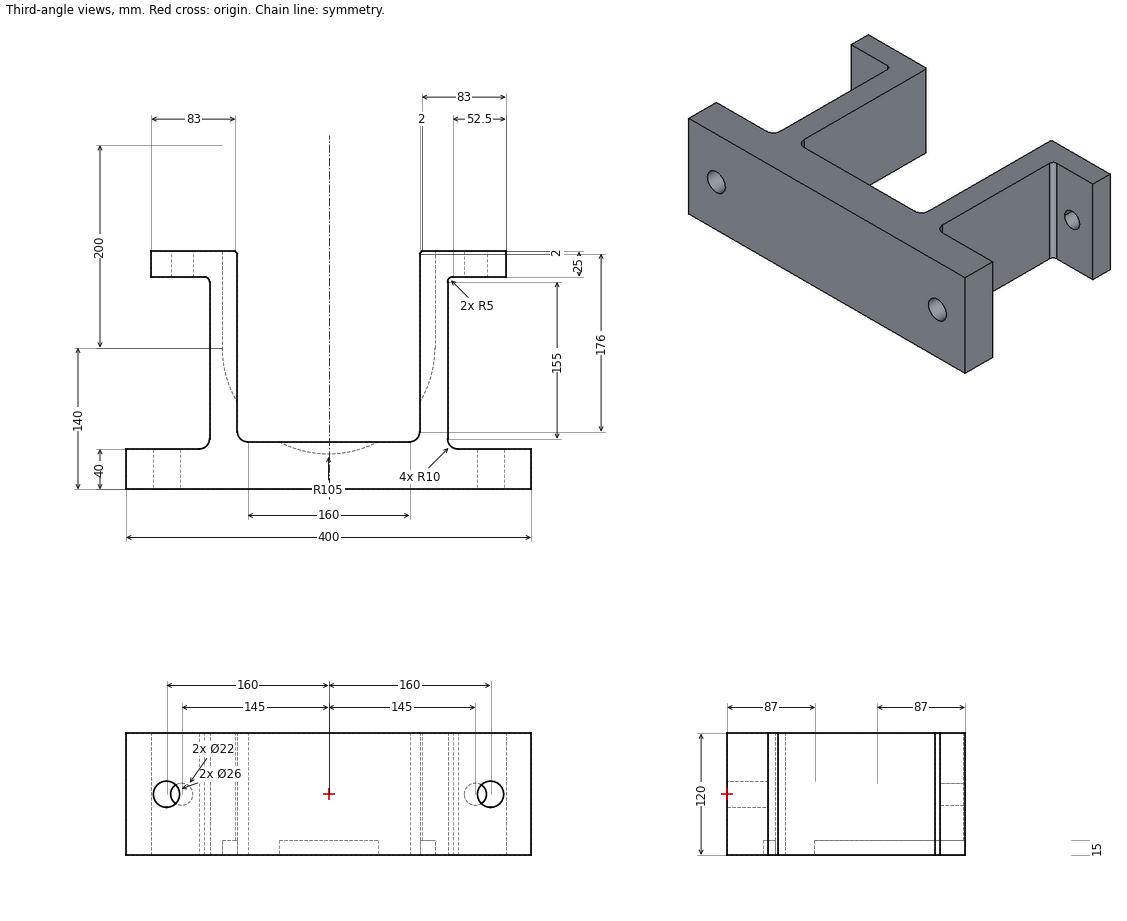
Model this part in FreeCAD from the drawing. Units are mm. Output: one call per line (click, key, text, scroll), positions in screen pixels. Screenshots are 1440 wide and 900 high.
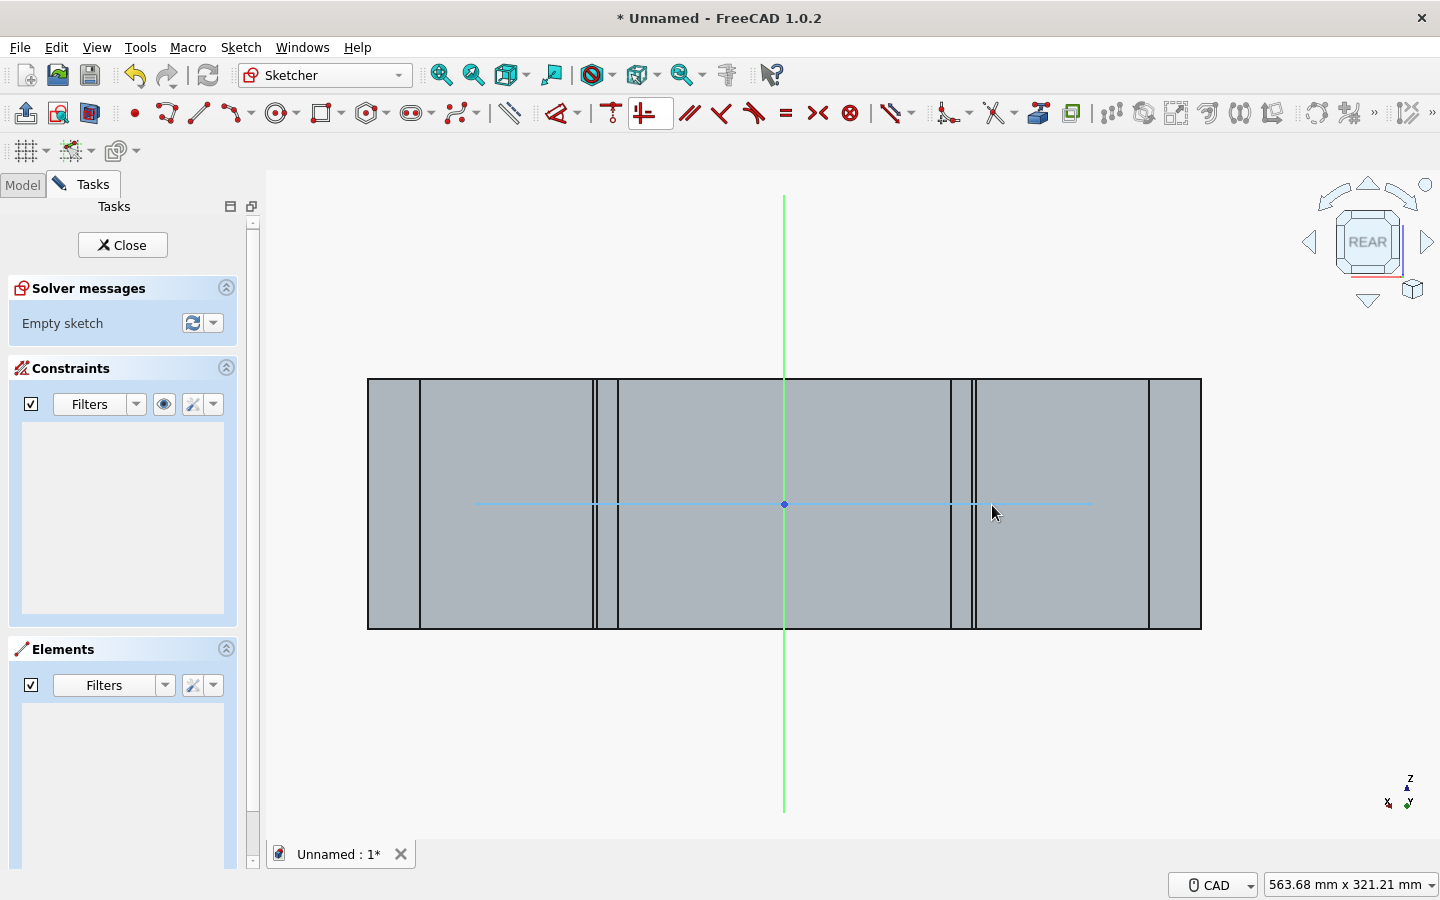
key(g)
key(c)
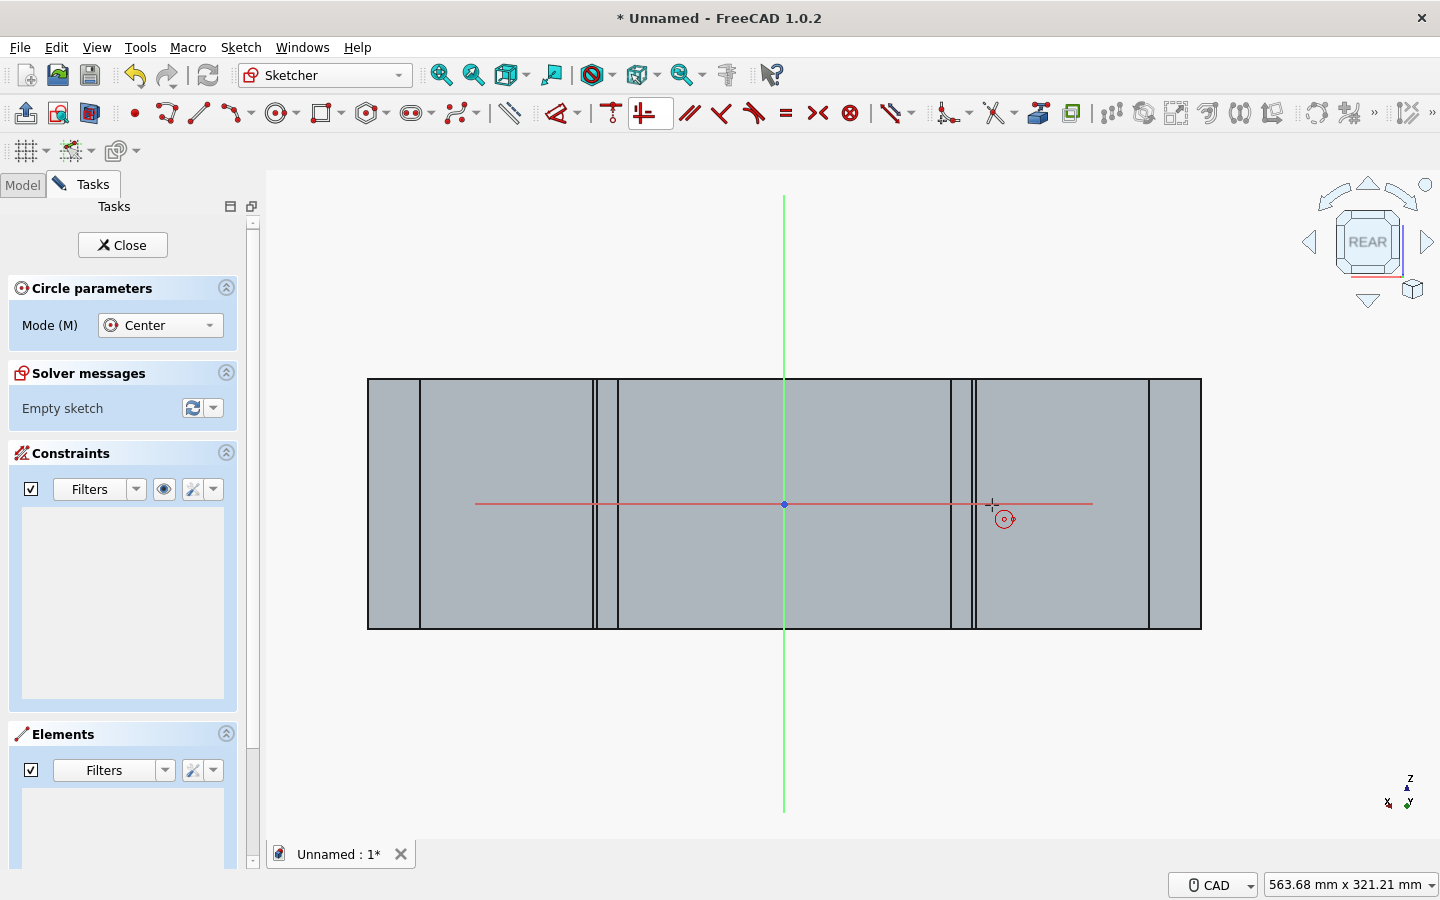
click(1086, 504)
move(1103, 488)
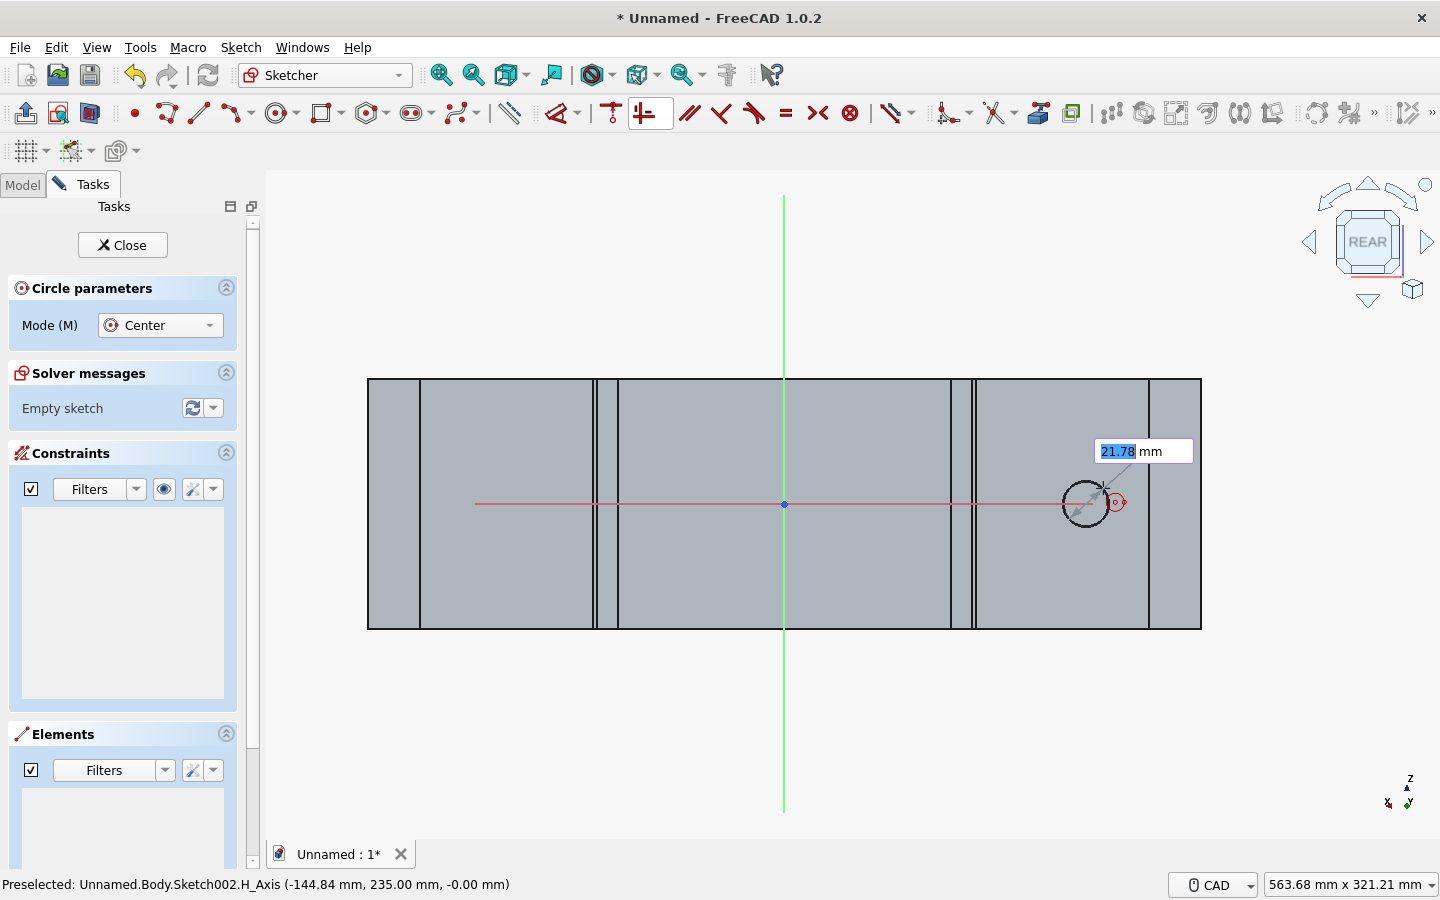
text(22)
key(Return)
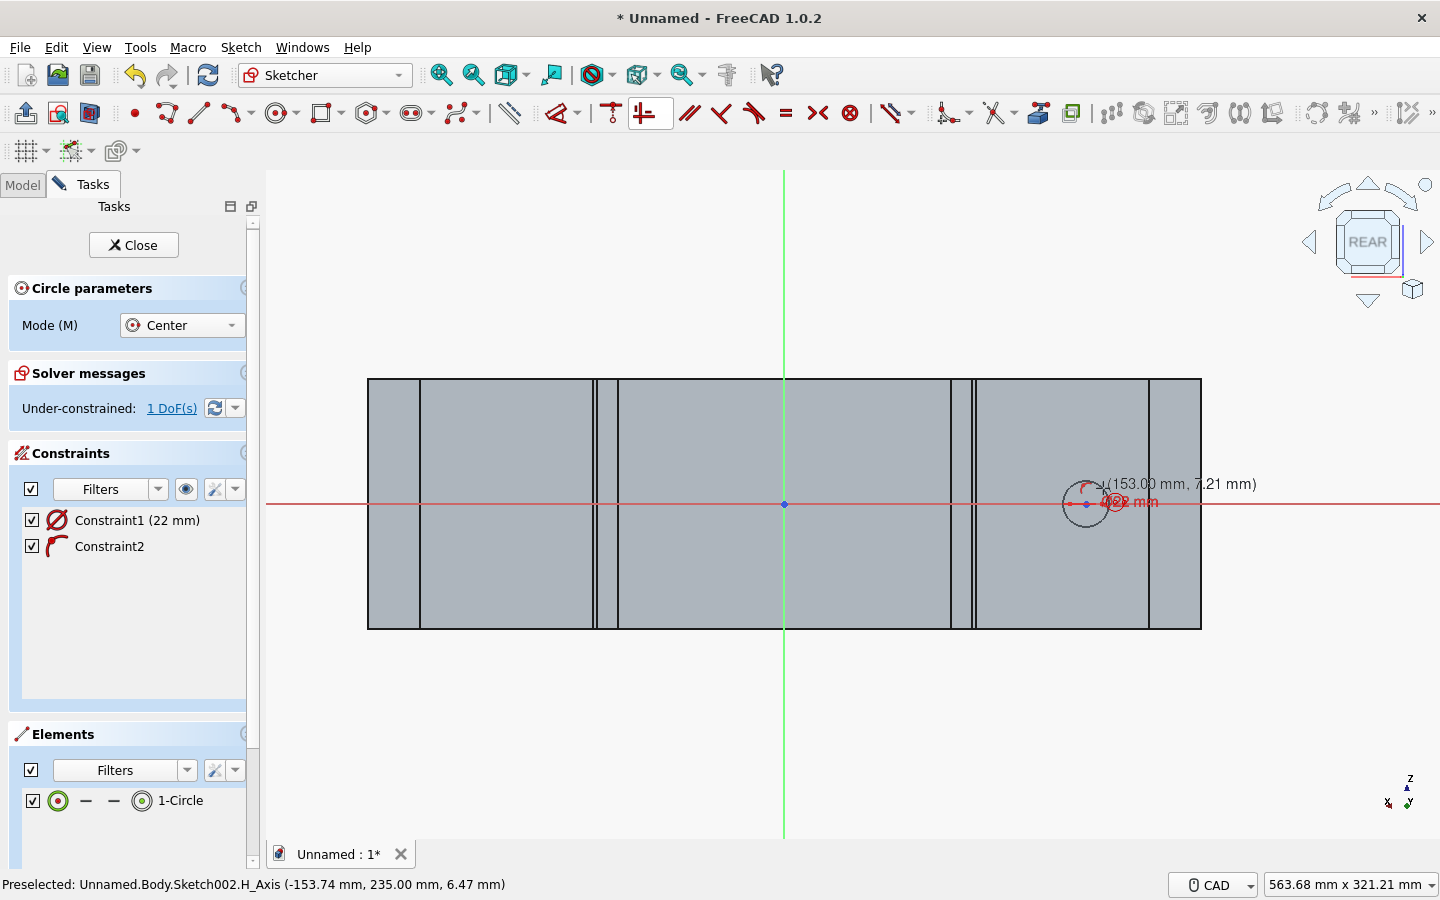
click(482, 504)
move(499, 488)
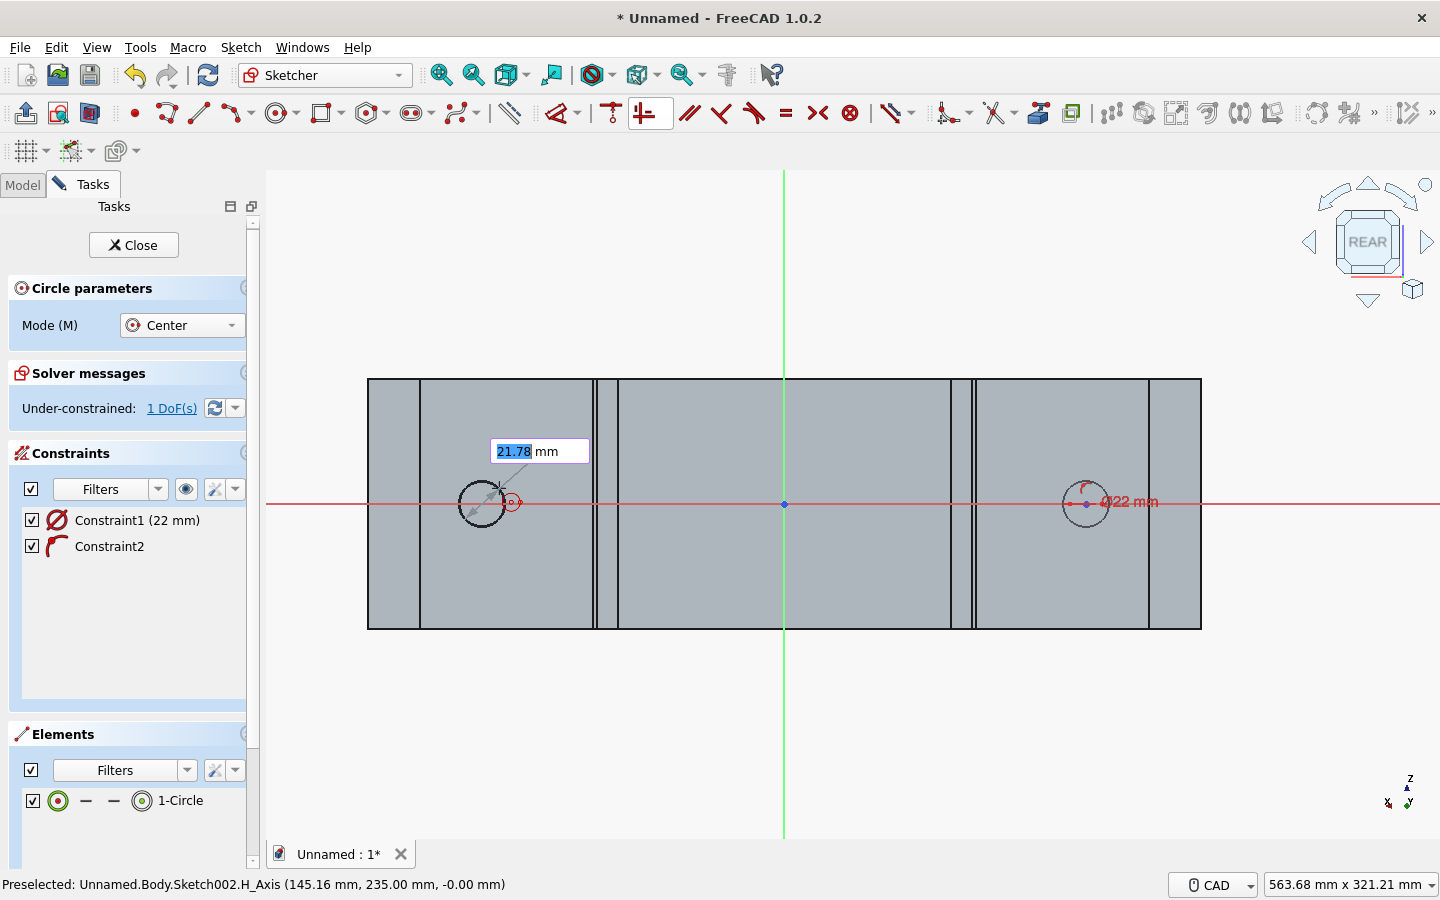
text(22)
key(Return)
key(Escape)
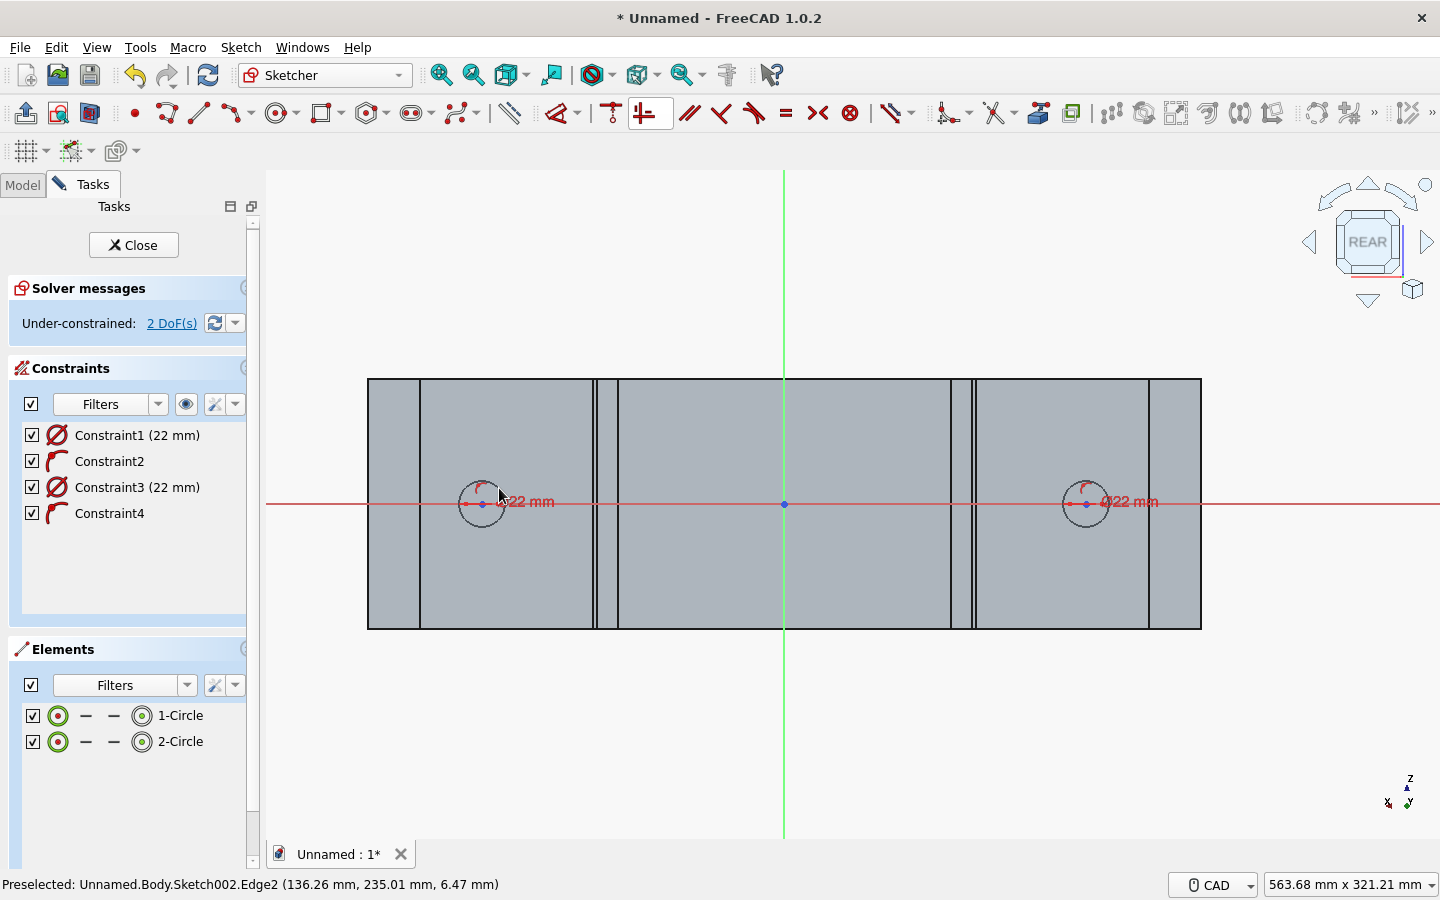
key(d)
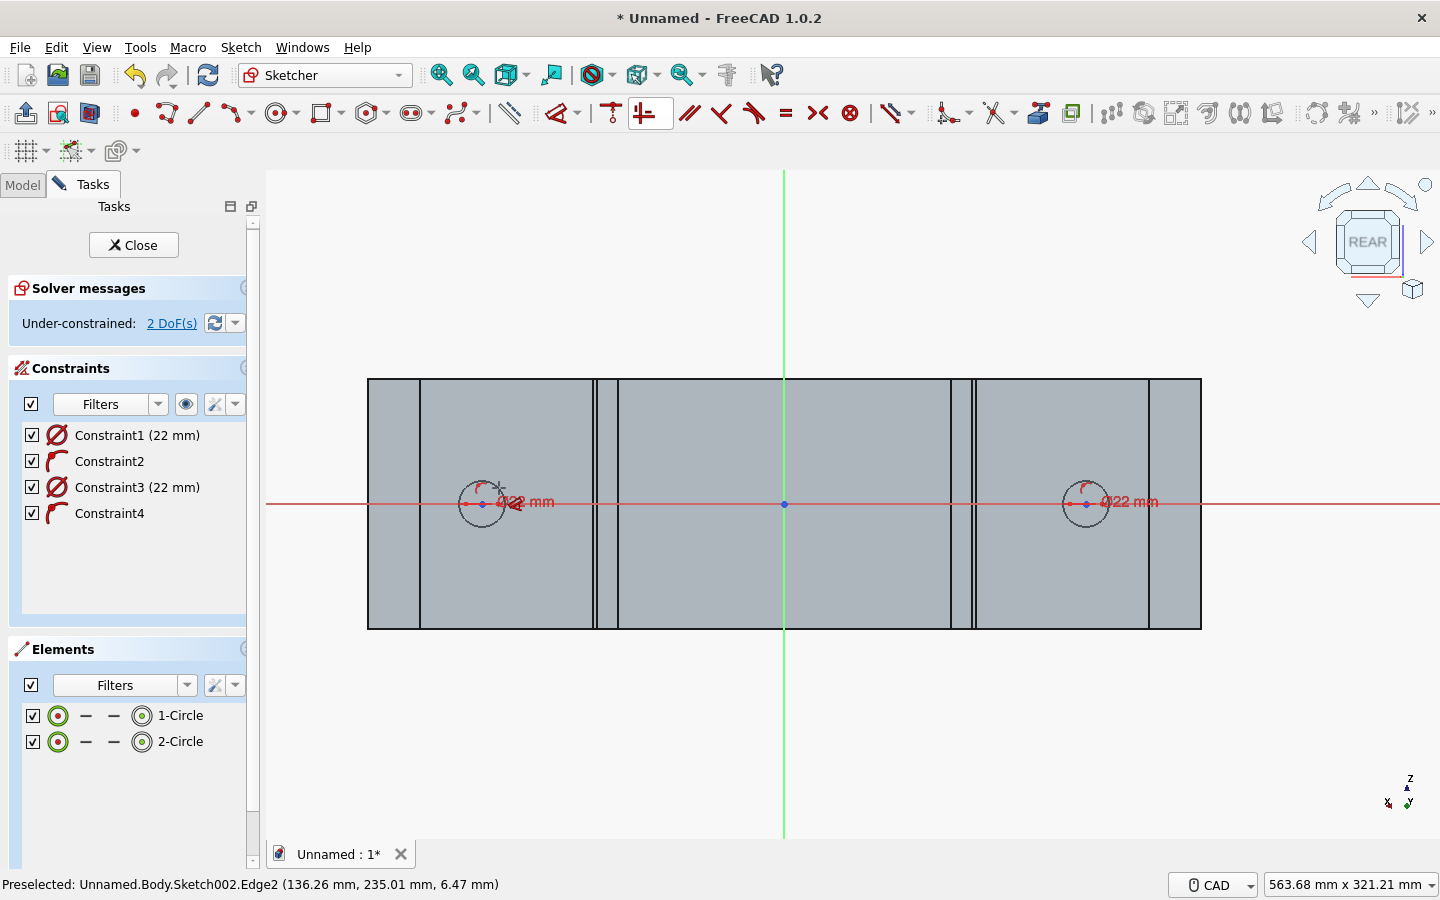
click(1086, 504)
click(935, 538)